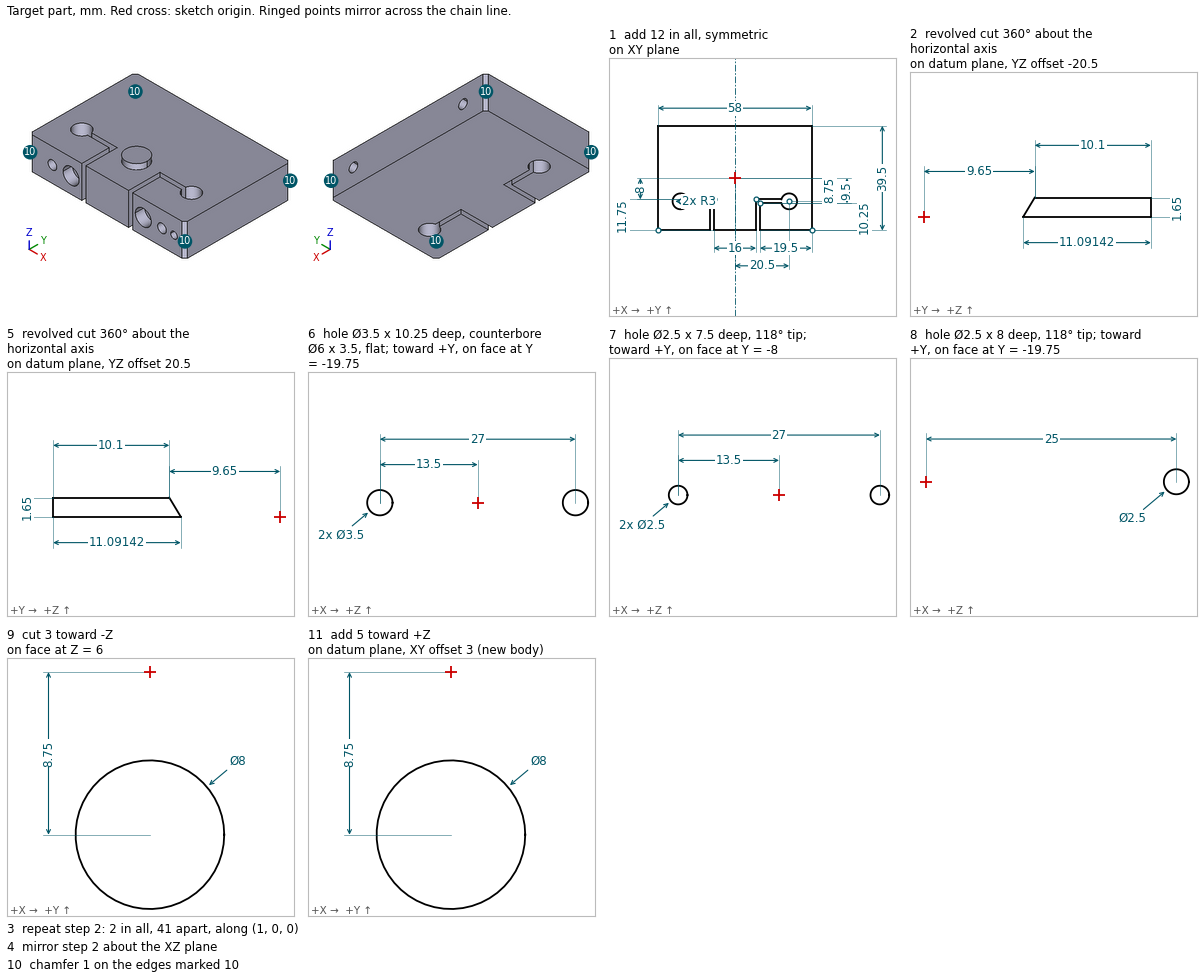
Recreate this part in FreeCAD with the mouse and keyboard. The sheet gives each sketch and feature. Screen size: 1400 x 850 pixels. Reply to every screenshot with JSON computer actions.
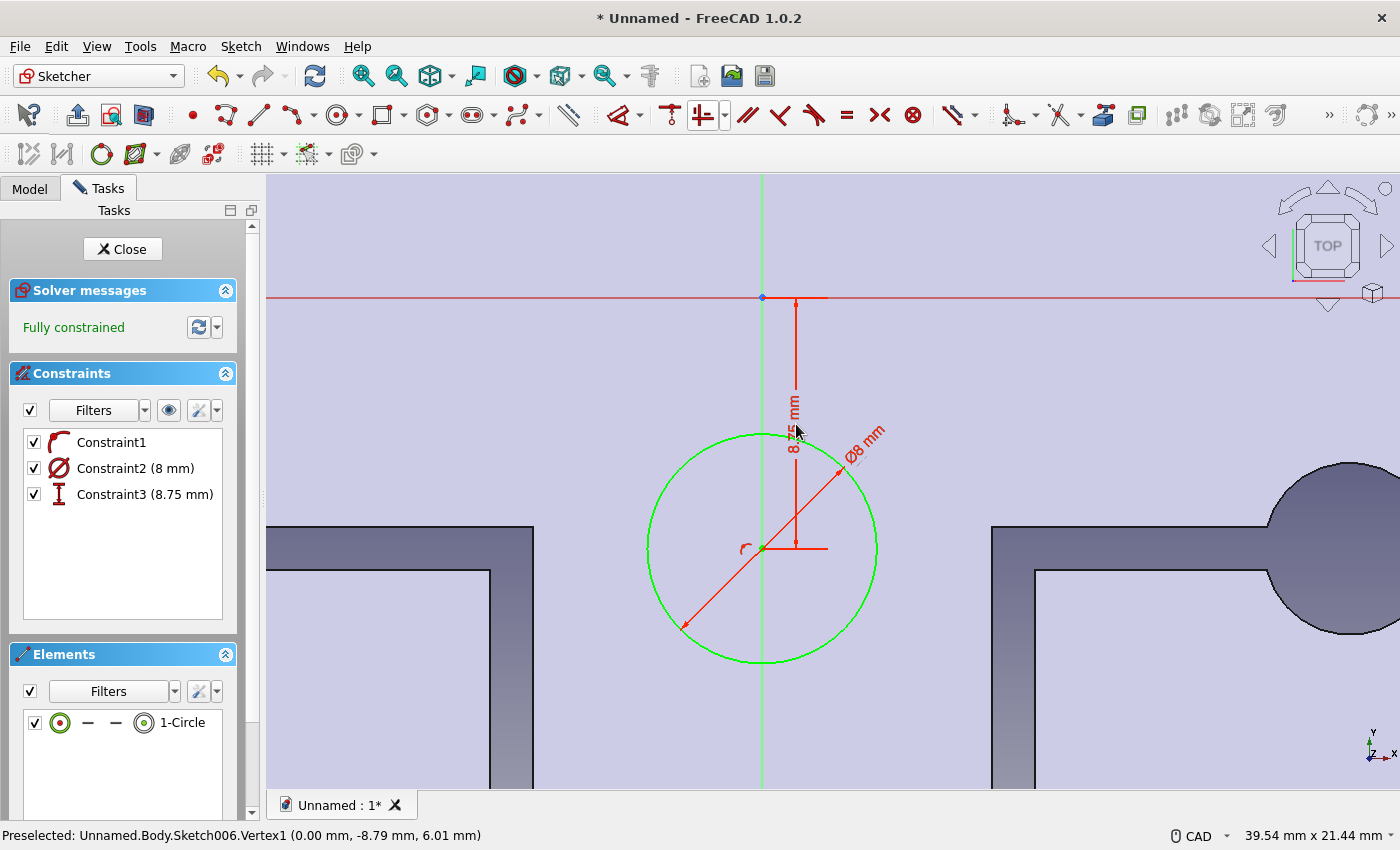
{"action": "left_click", "coordinate": [123, 249]}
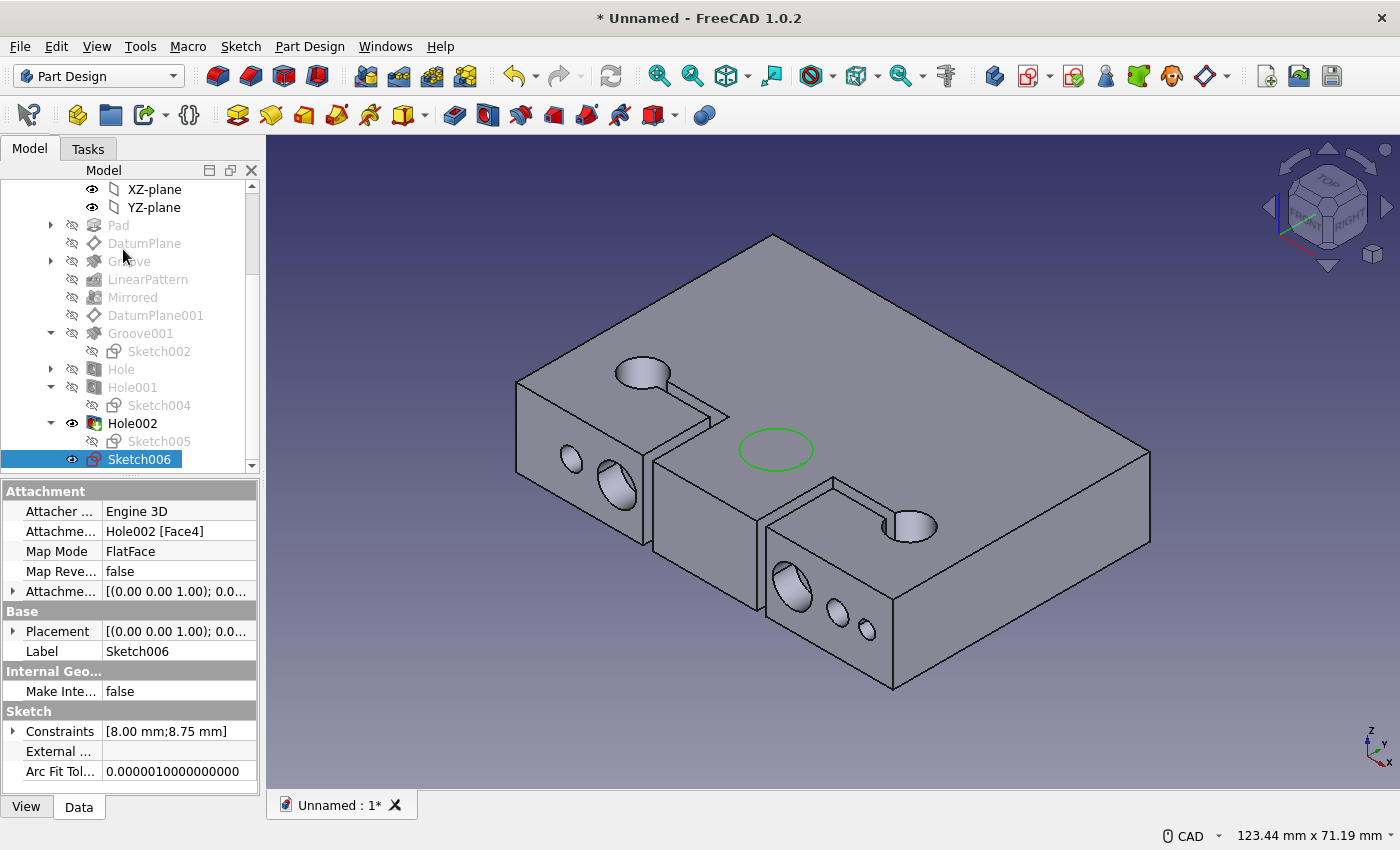
{"action": "left_click", "coordinate": [455, 116]}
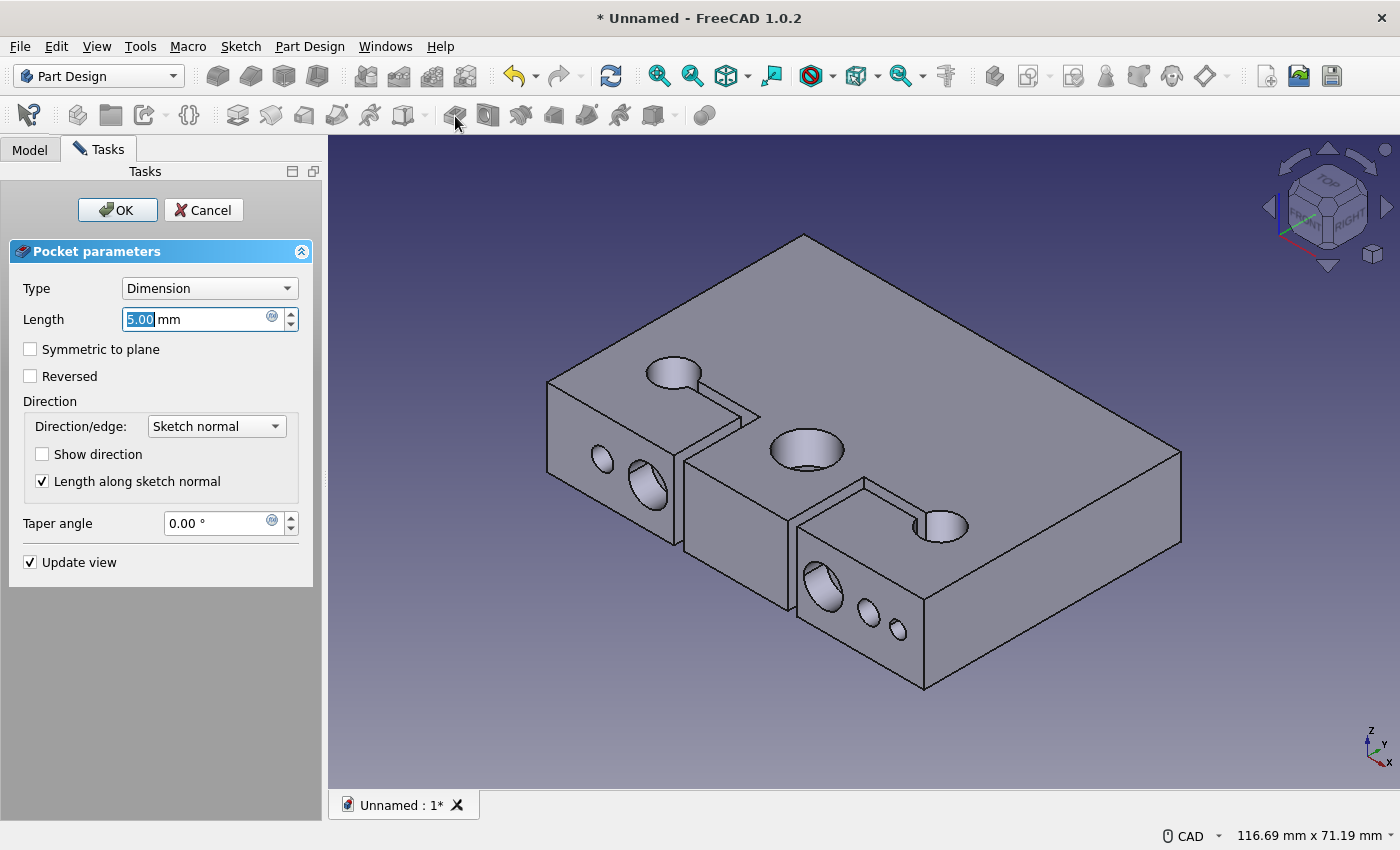
{"action": "type", "text": "3"}
{"action": "key", "text": "Tab"}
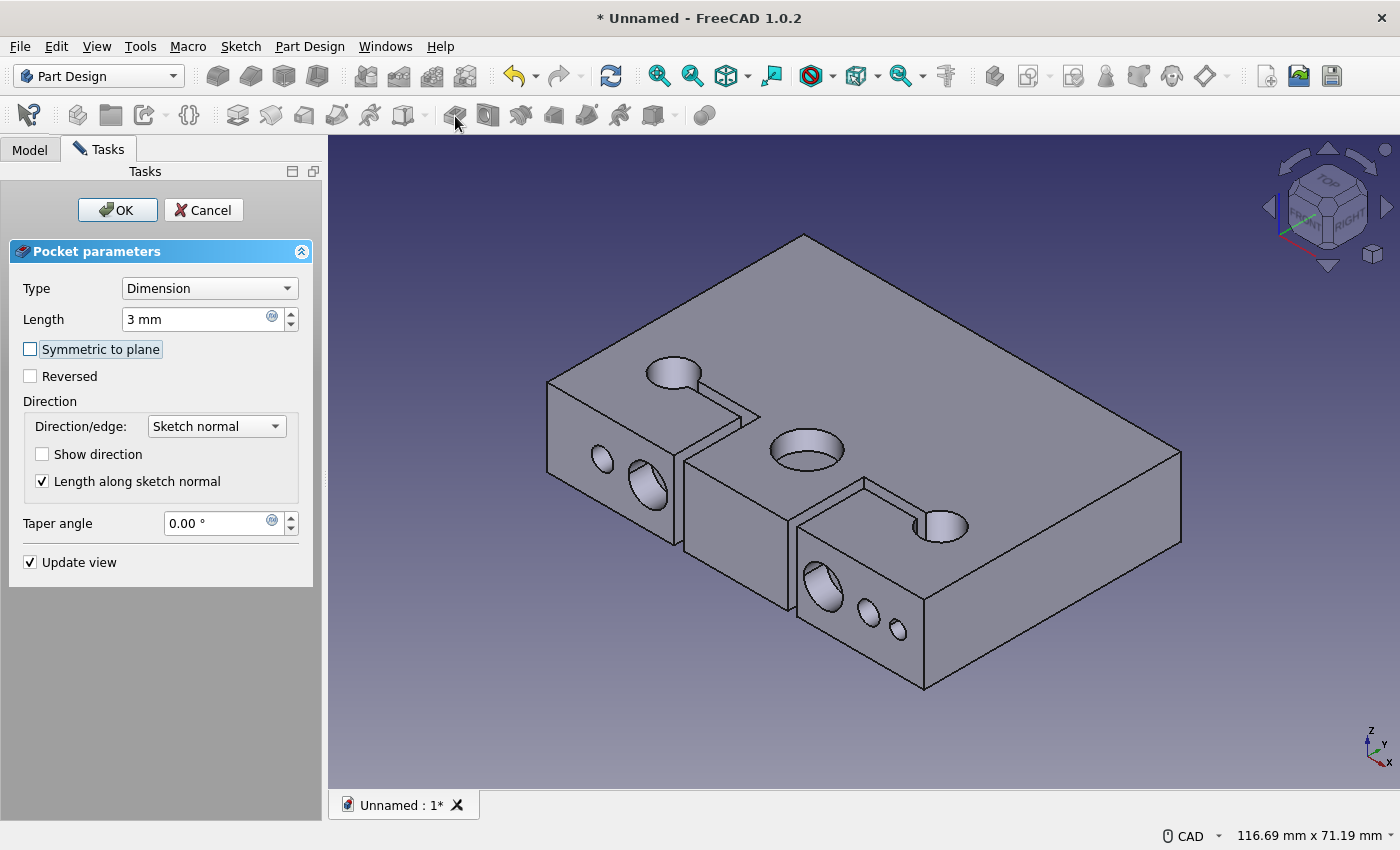
{"action": "left_click", "coordinate": [118, 210]}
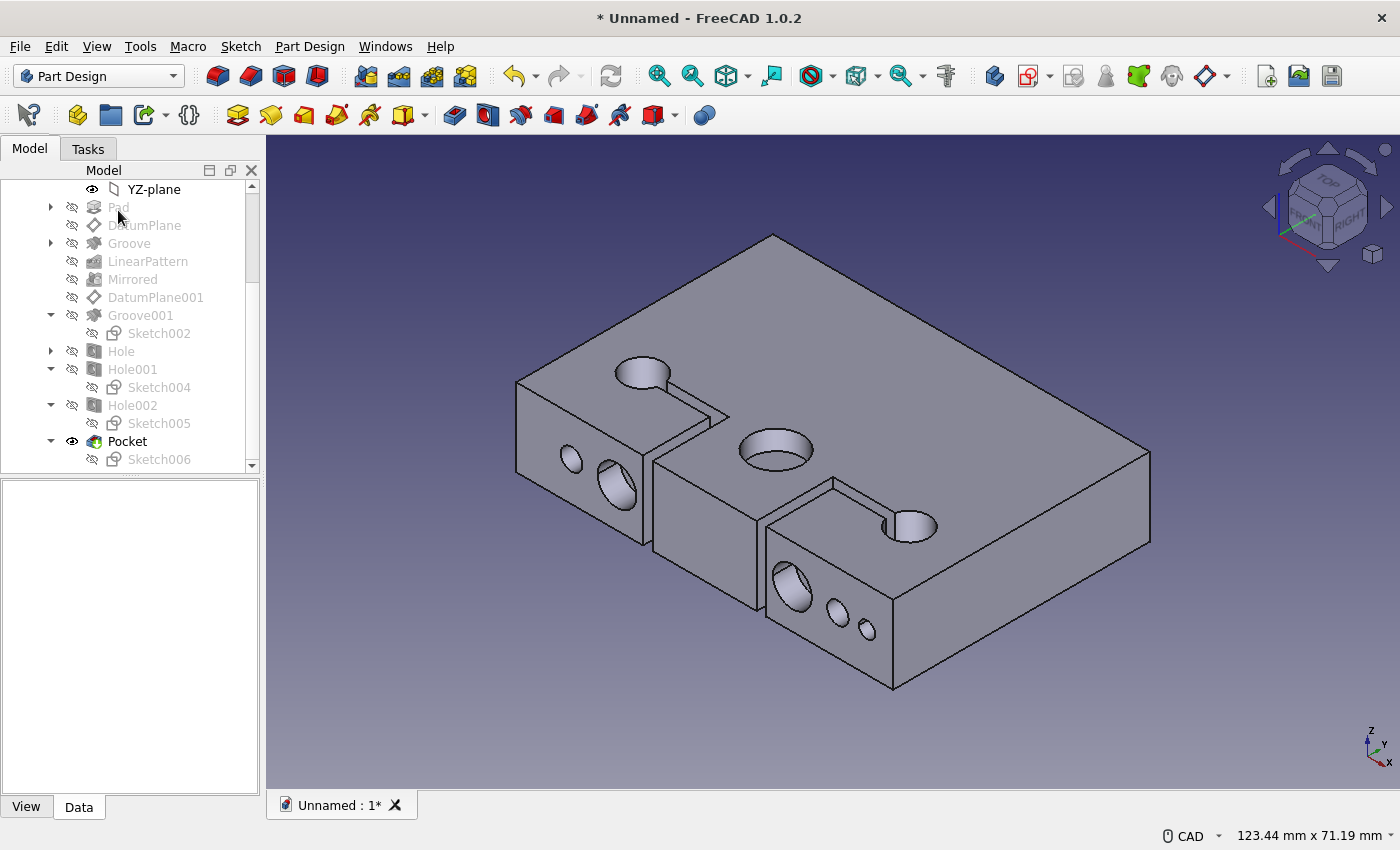
{"action": "left_click", "coordinate": [893, 644]}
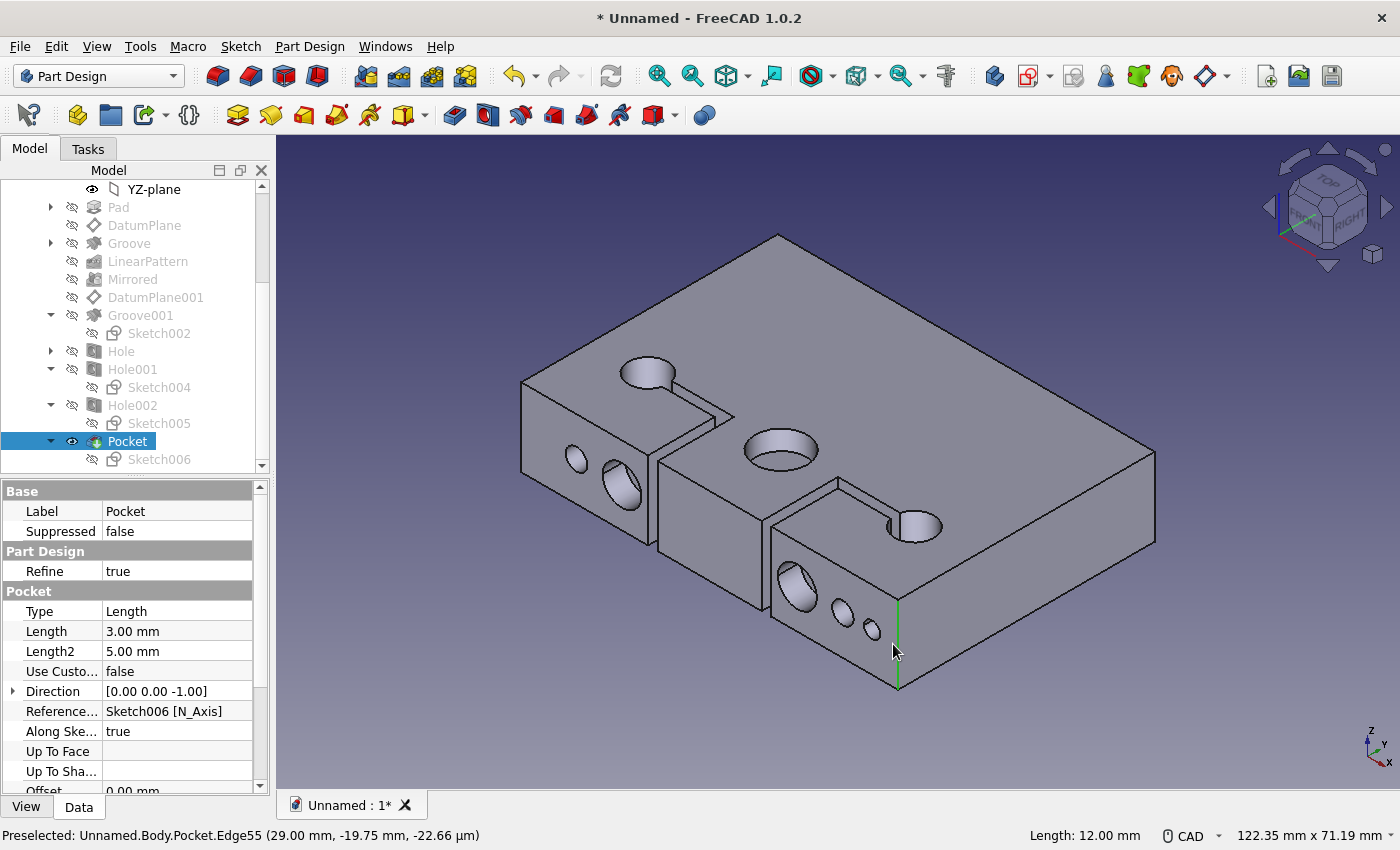
{"action": "key", "text": "2"}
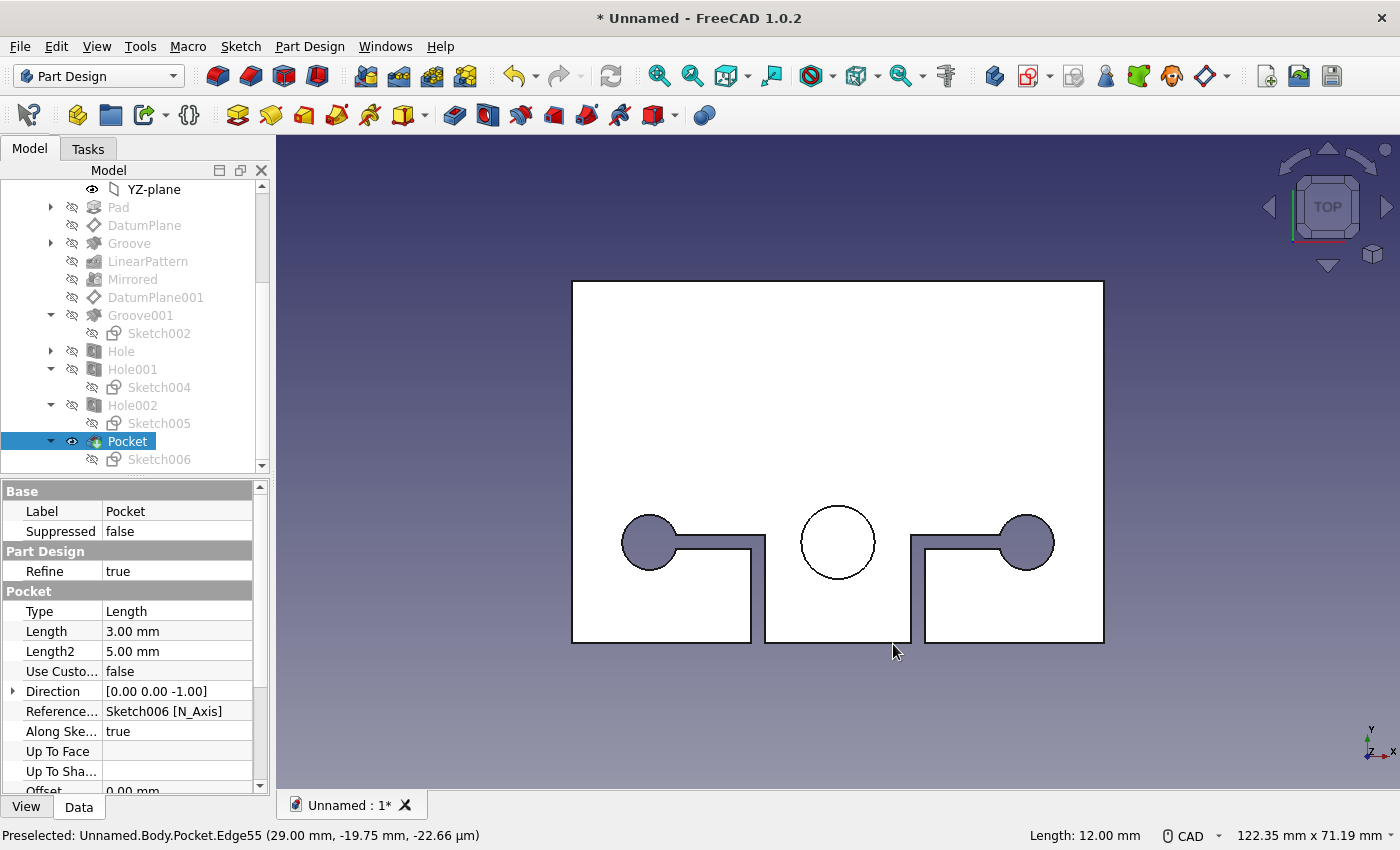
{"action": "key", "text": "0"}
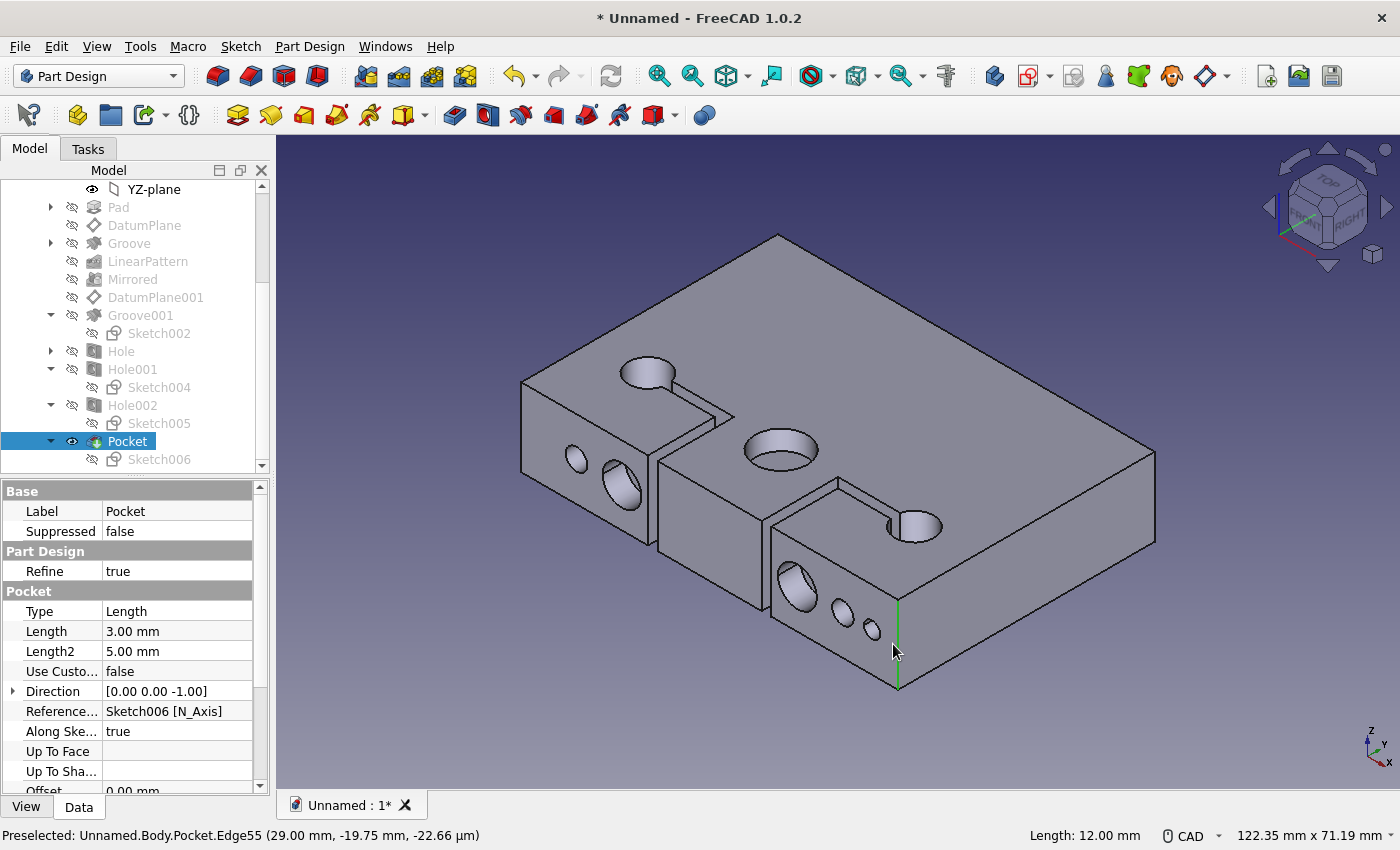
{"action": "key", "text": "1"}